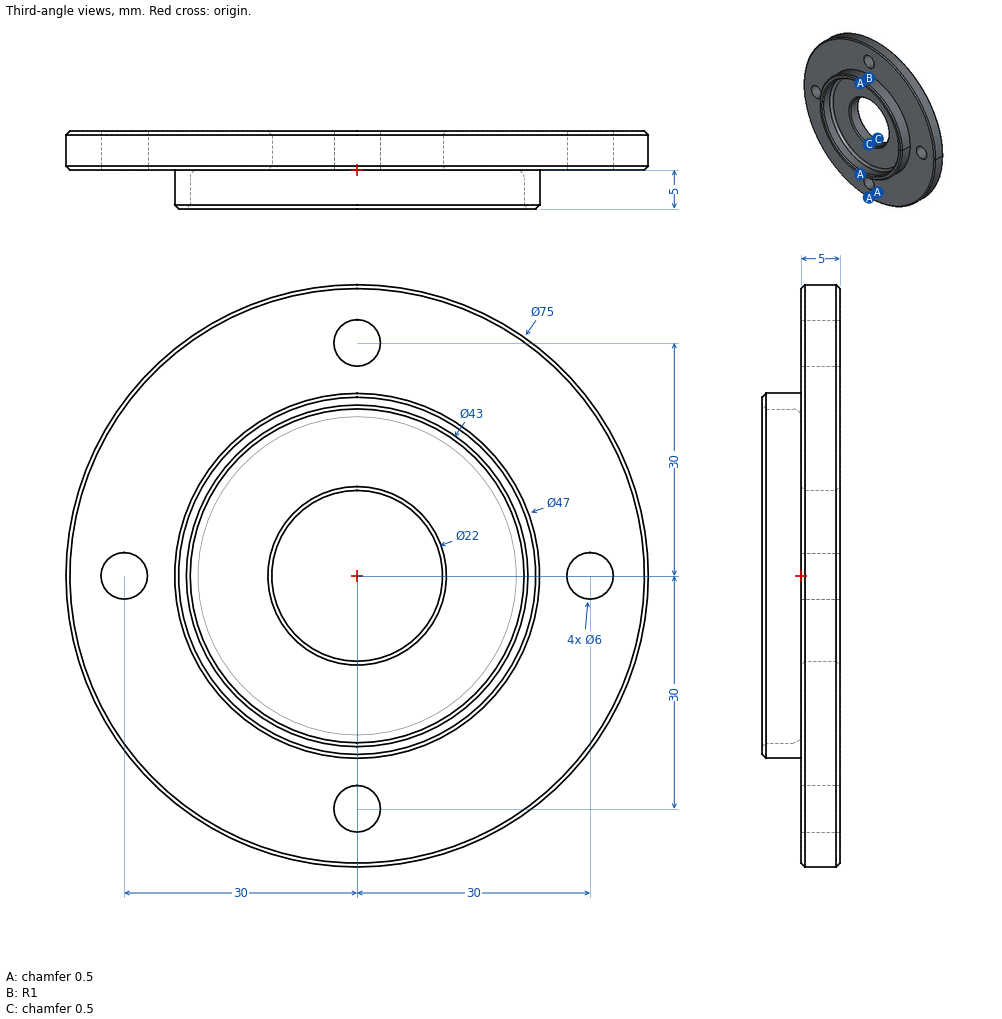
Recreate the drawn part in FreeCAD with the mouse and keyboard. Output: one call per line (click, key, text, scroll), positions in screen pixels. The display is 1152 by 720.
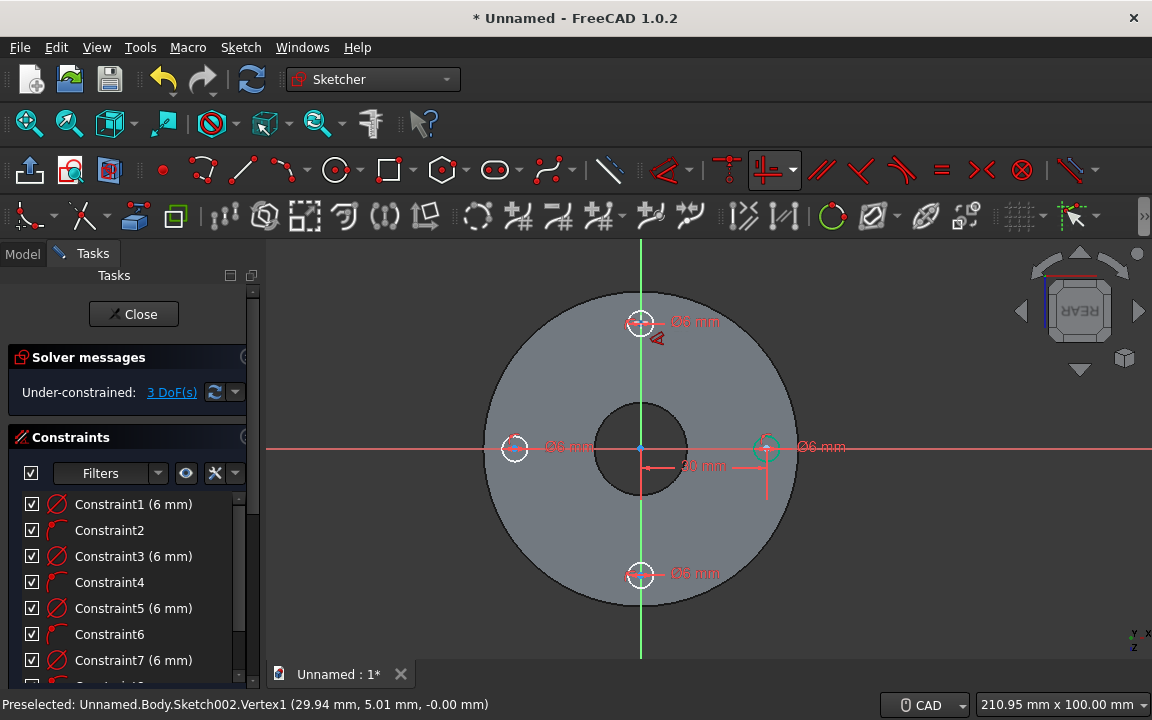
click(641, 575)
click(675, 512)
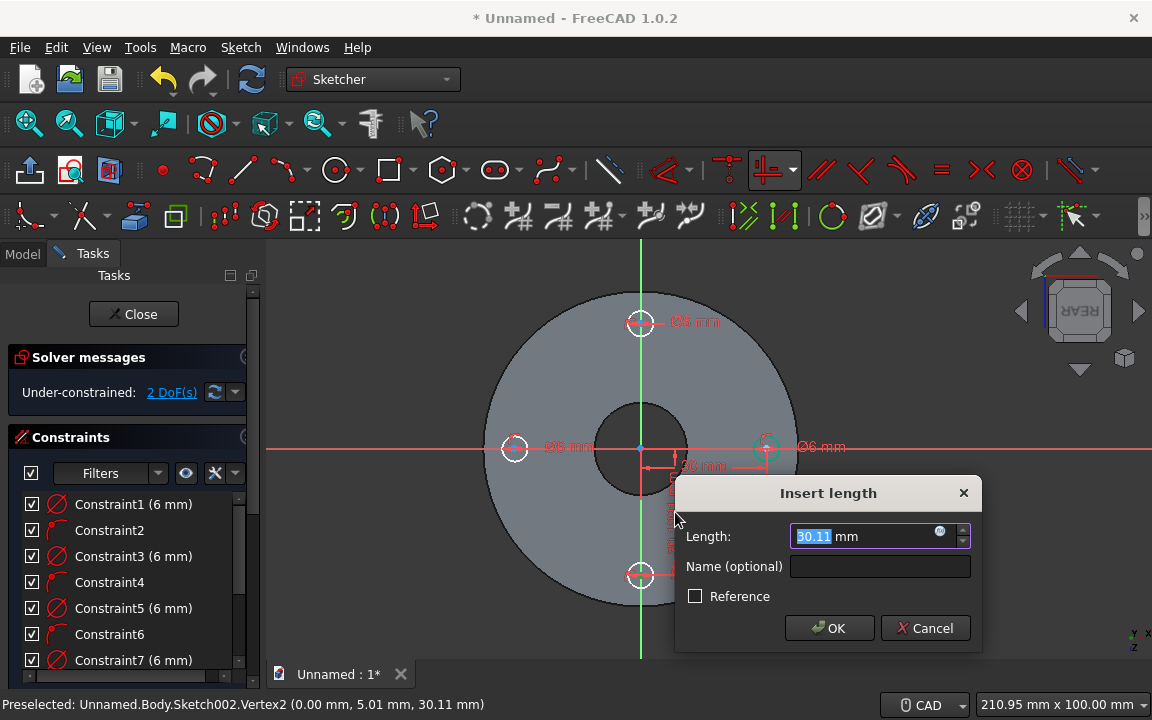
text(30)
key(Return)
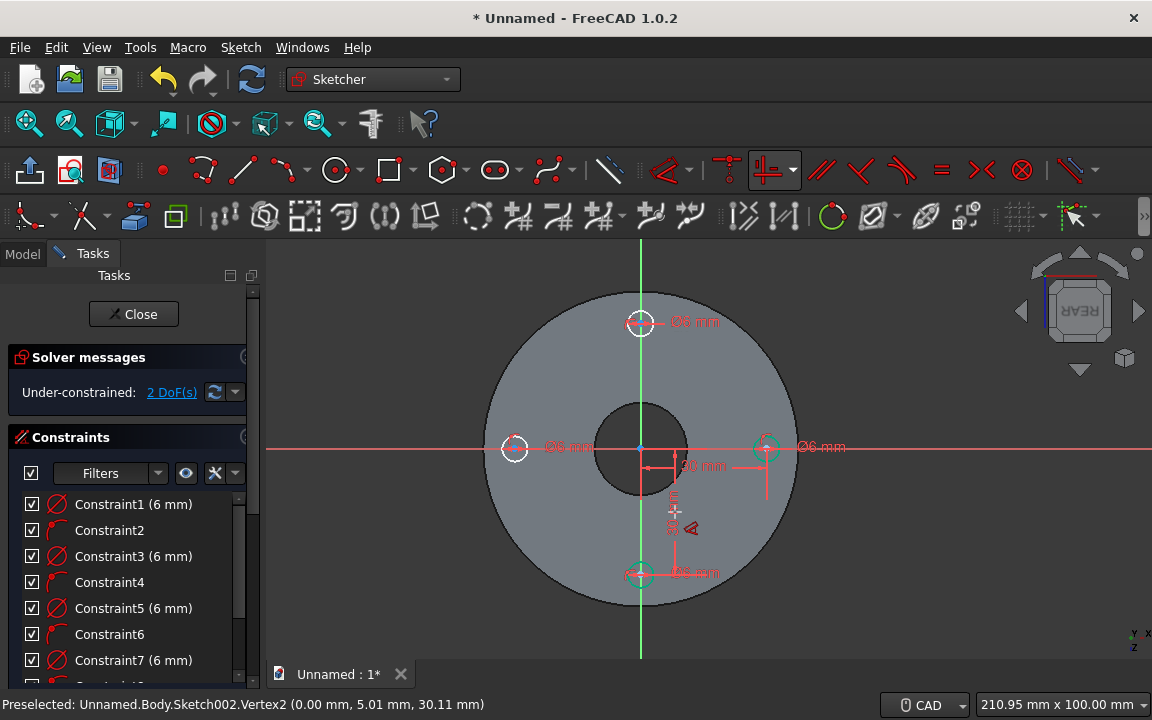
click(515, 449)
click(578, 483)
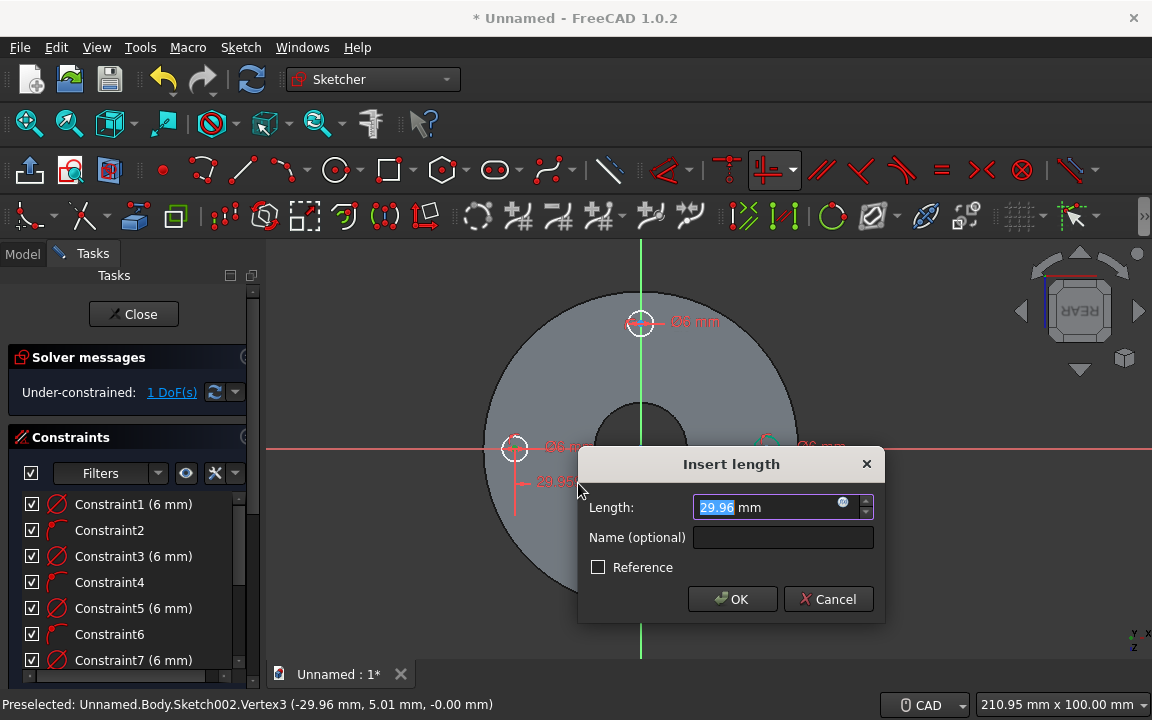
text(30)
key(Return)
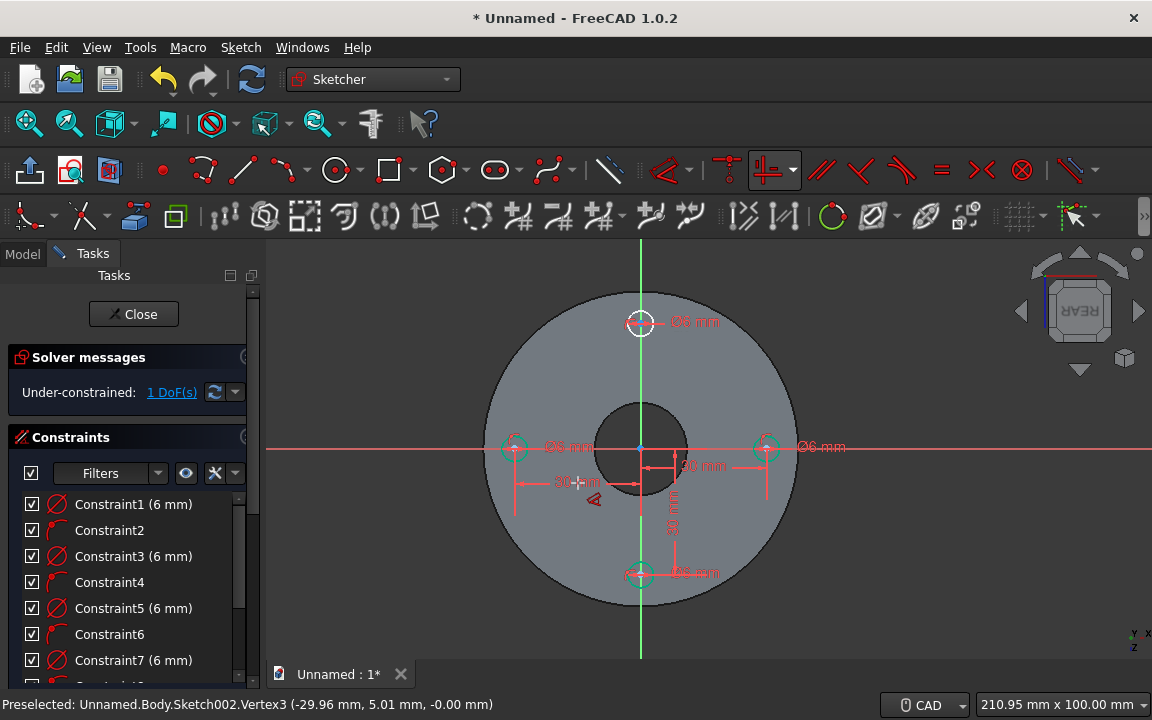
click(641, 324)
click(675, 386)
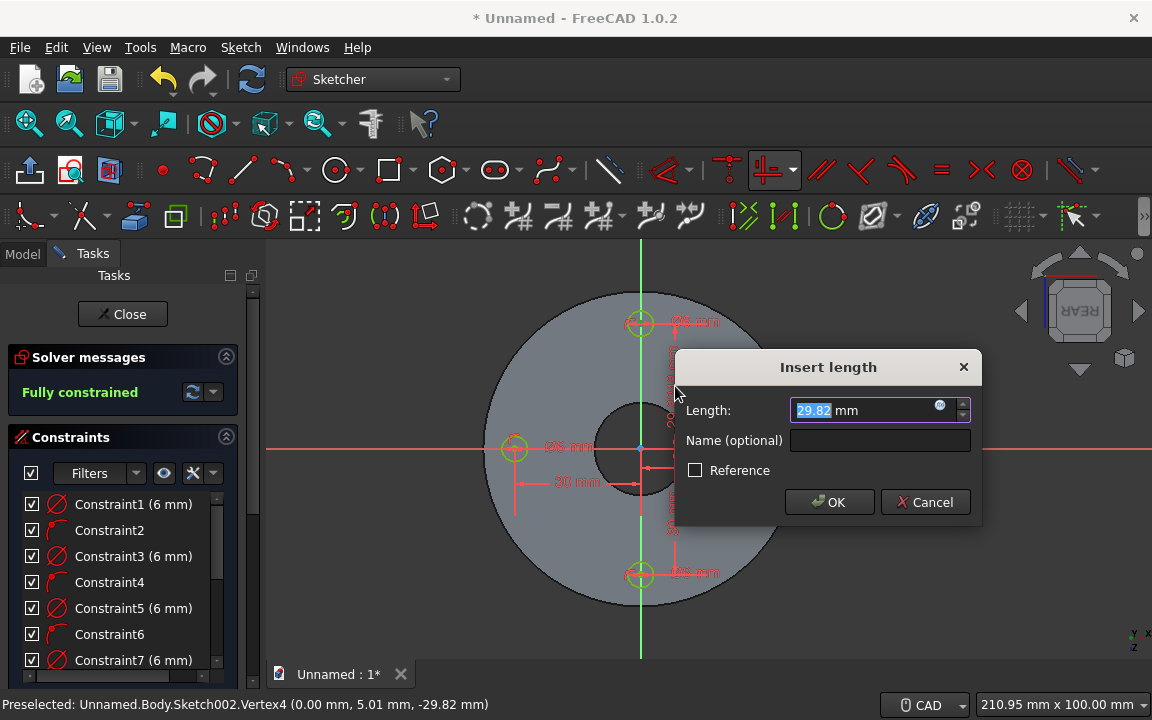
text(30)
key(Return)
key(Escape)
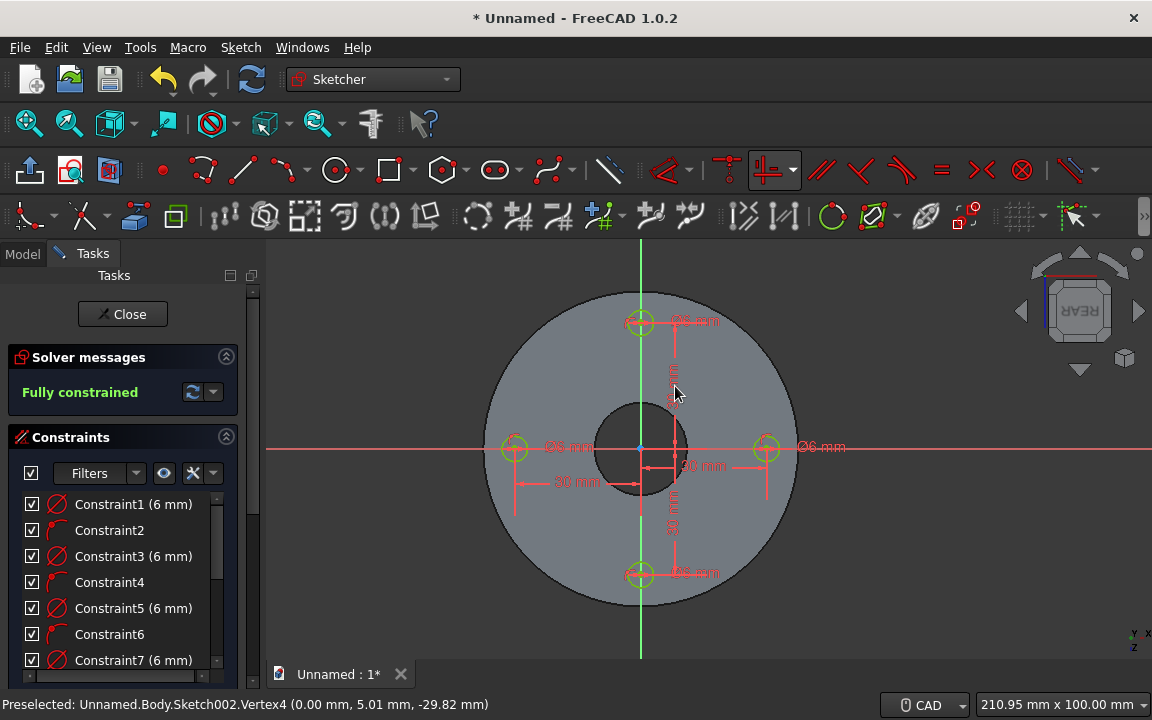
click(123, 314)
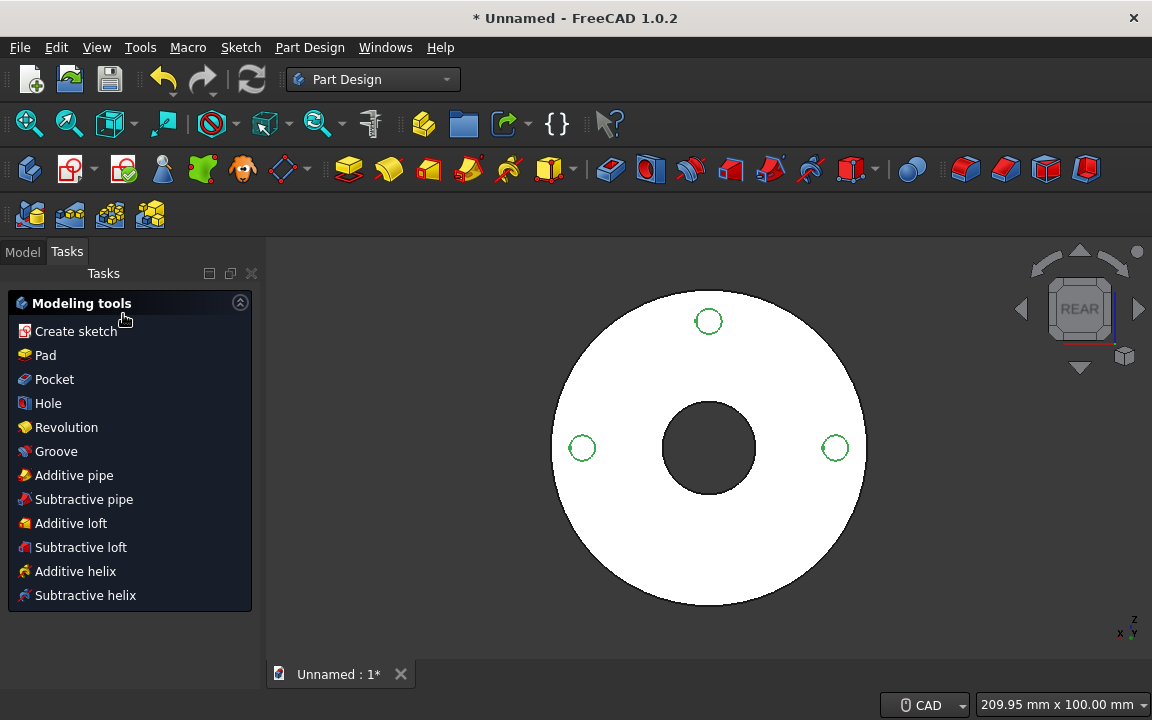
click(612, 170)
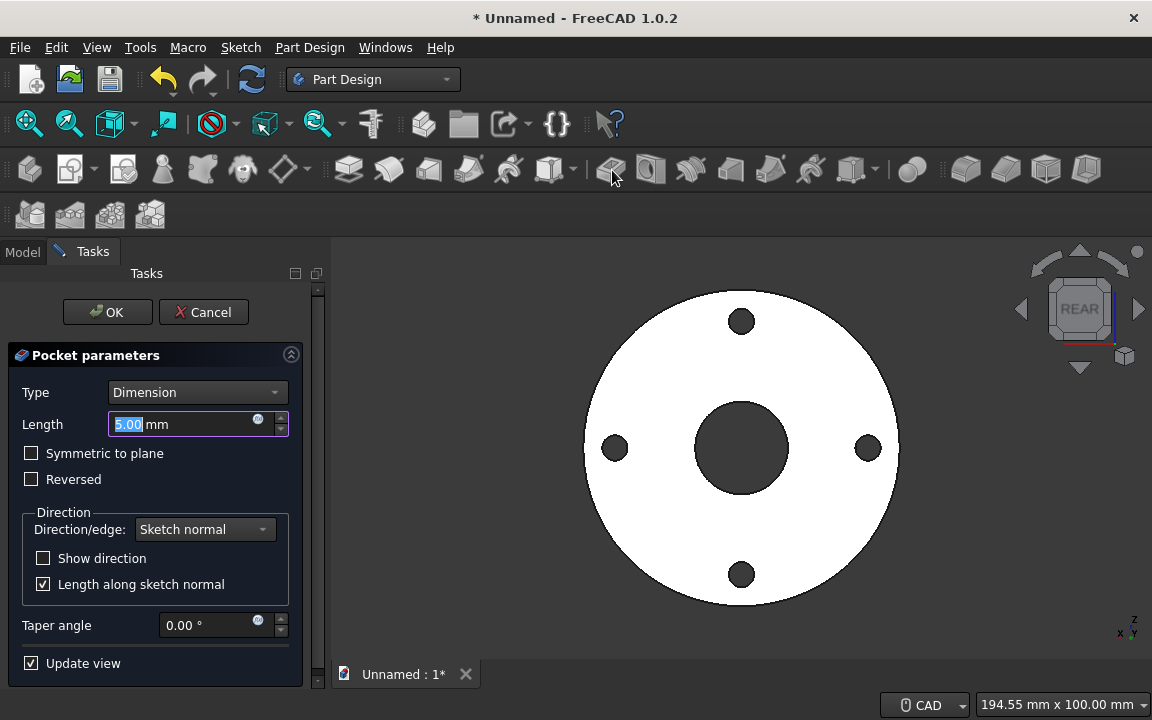
click(198, 392)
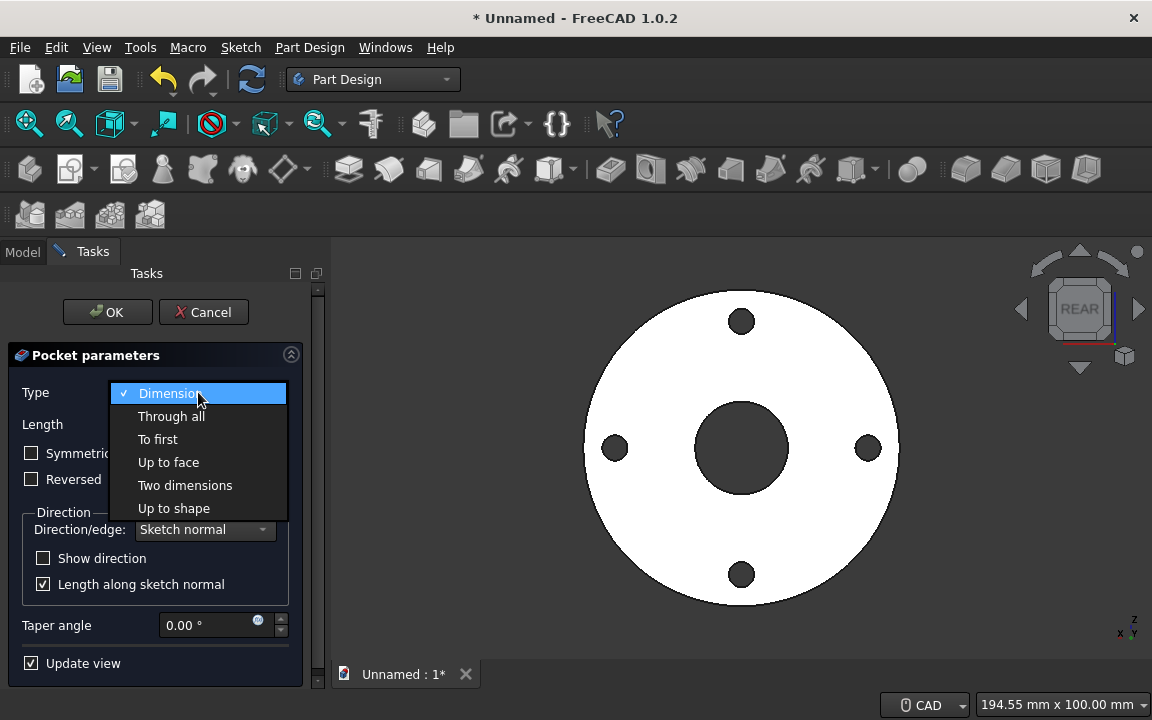
click(198, 416)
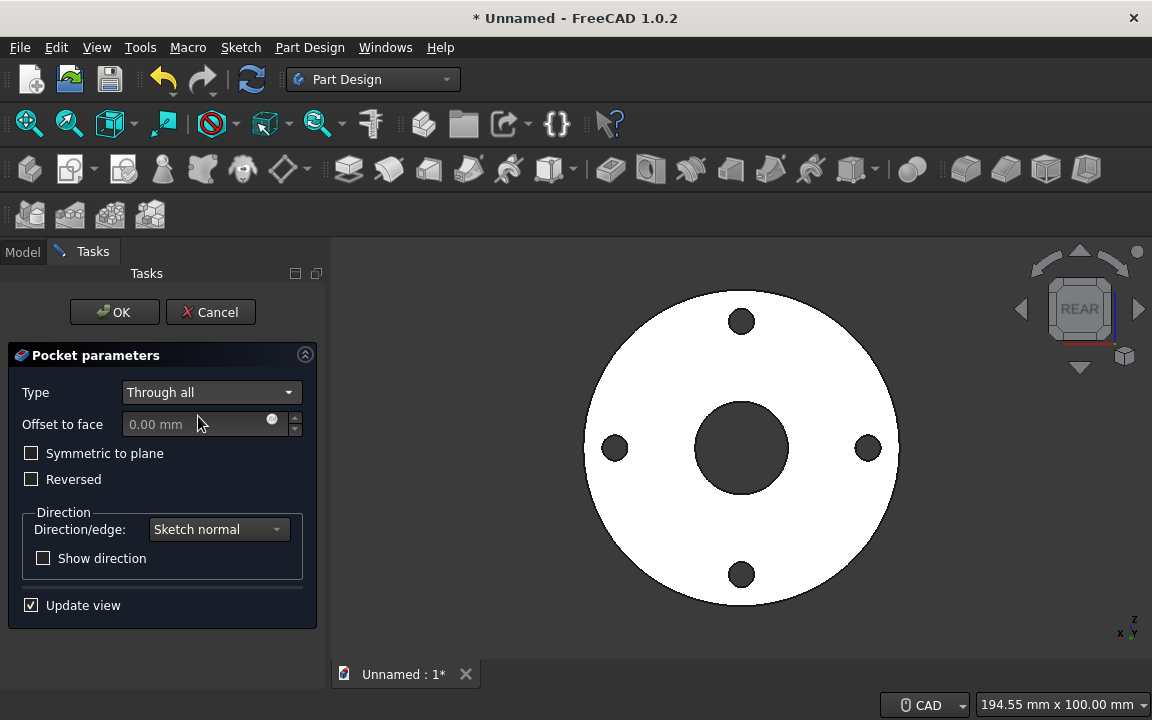
click(115, 312)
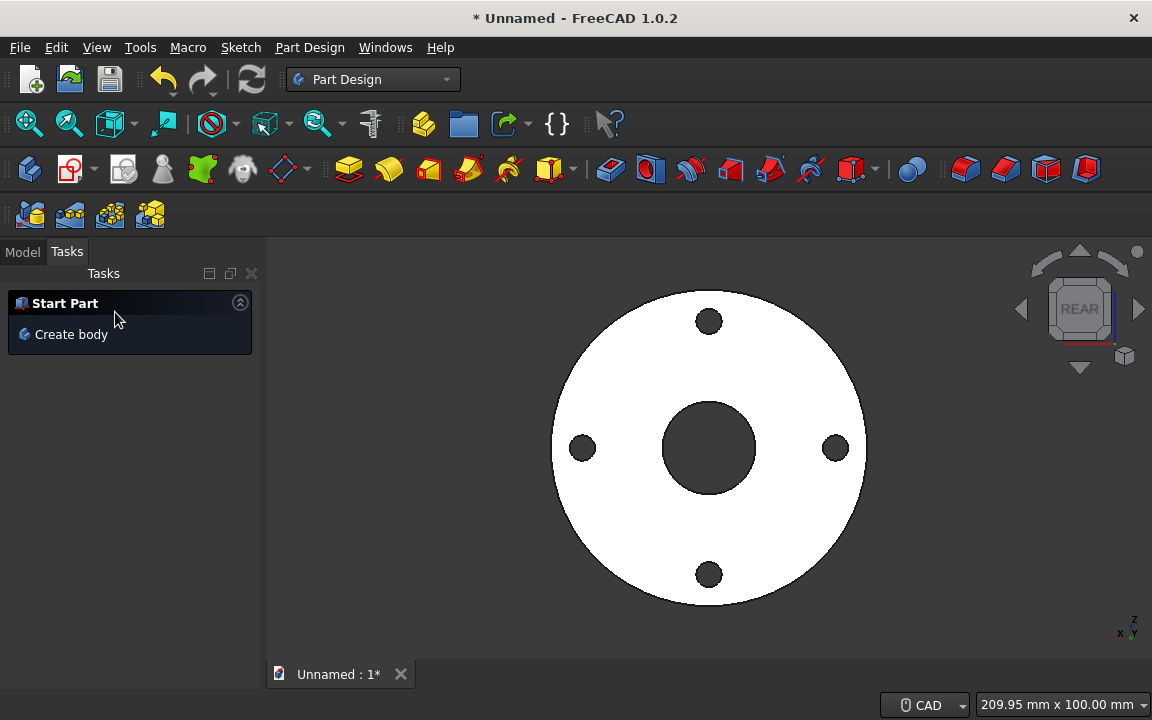
click(867, 447)